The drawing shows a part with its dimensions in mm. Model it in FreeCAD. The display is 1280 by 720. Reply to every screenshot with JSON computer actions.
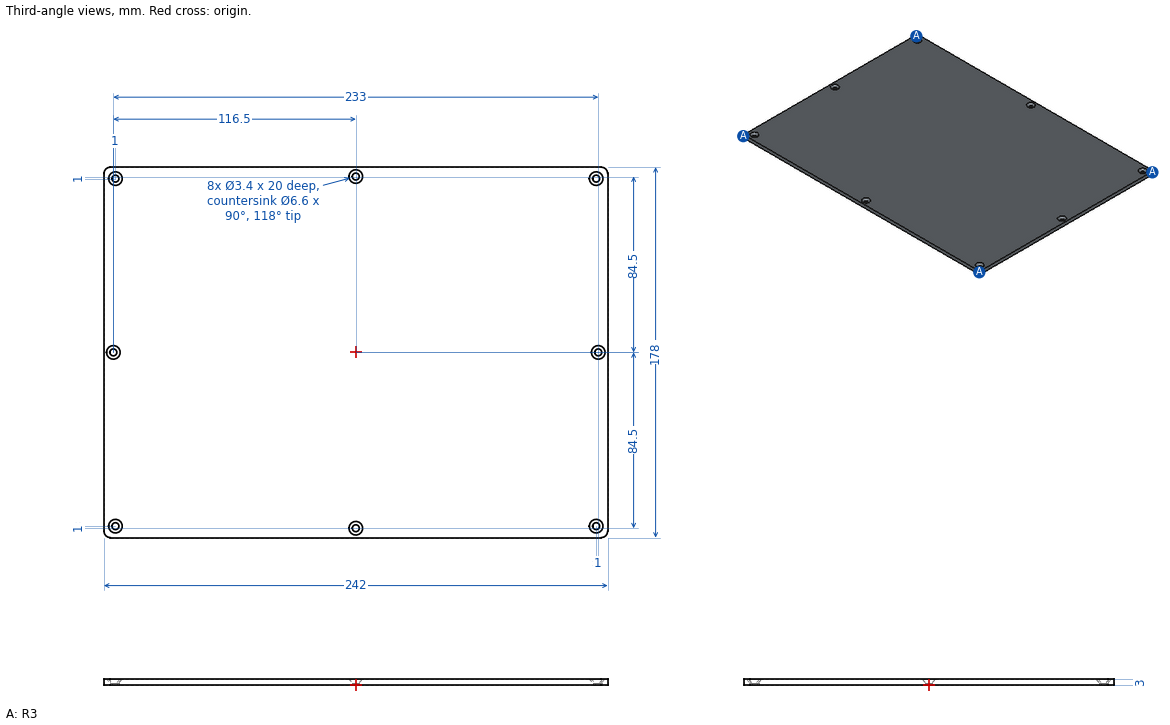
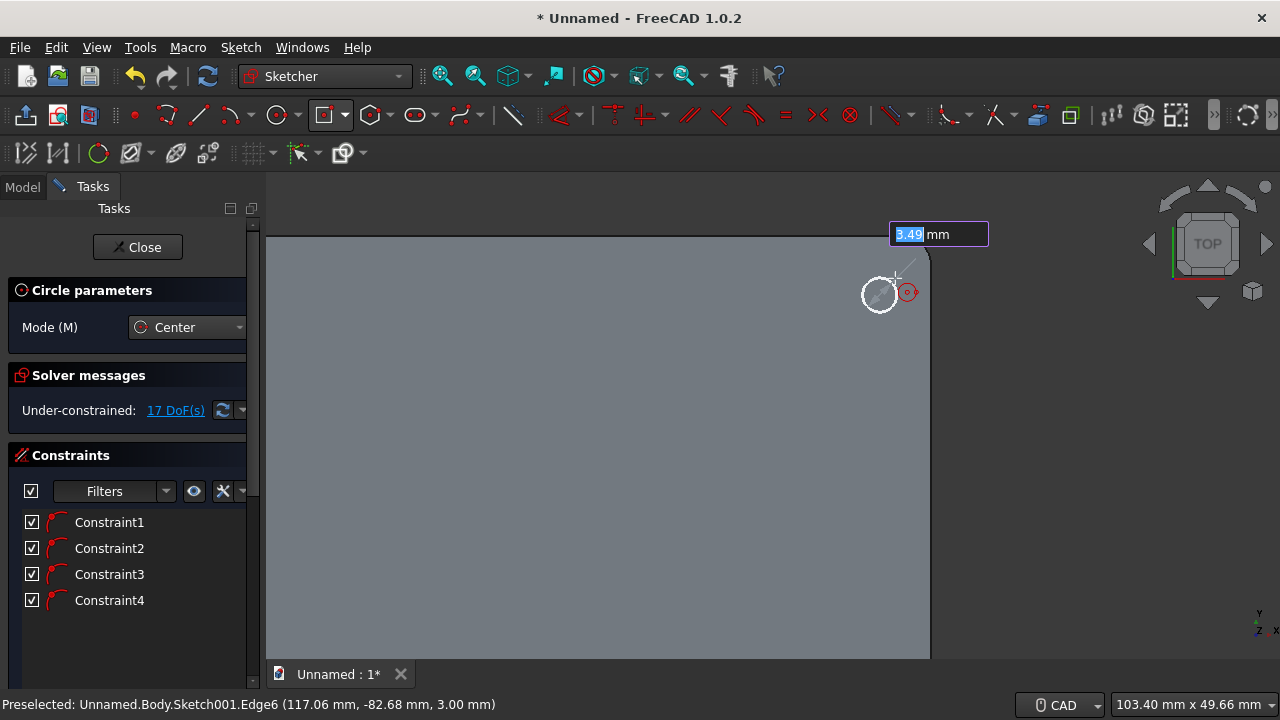
{"action": "left_click", "coordinate": [889, 278]}
{"action": "key", "text": "Escape"}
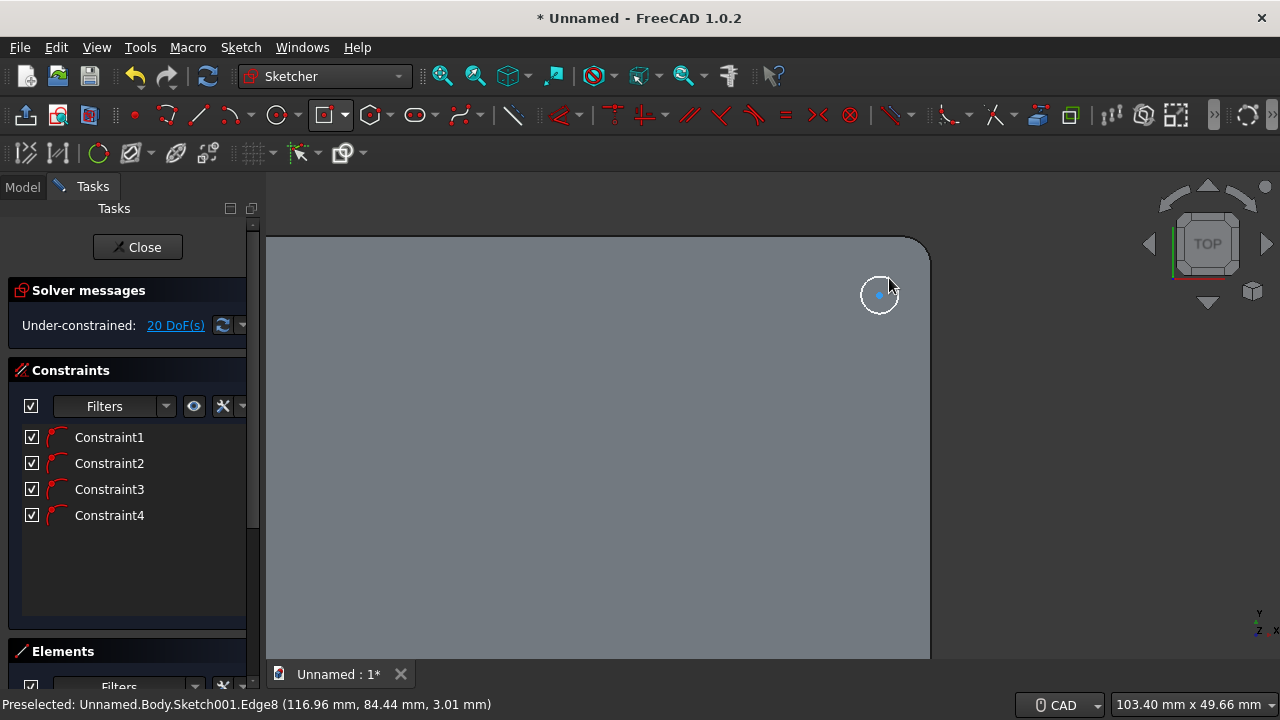
{"action": "scroll", "coordinate": [895, 278], "scroll_direction": "down", "scroll_amount": 9}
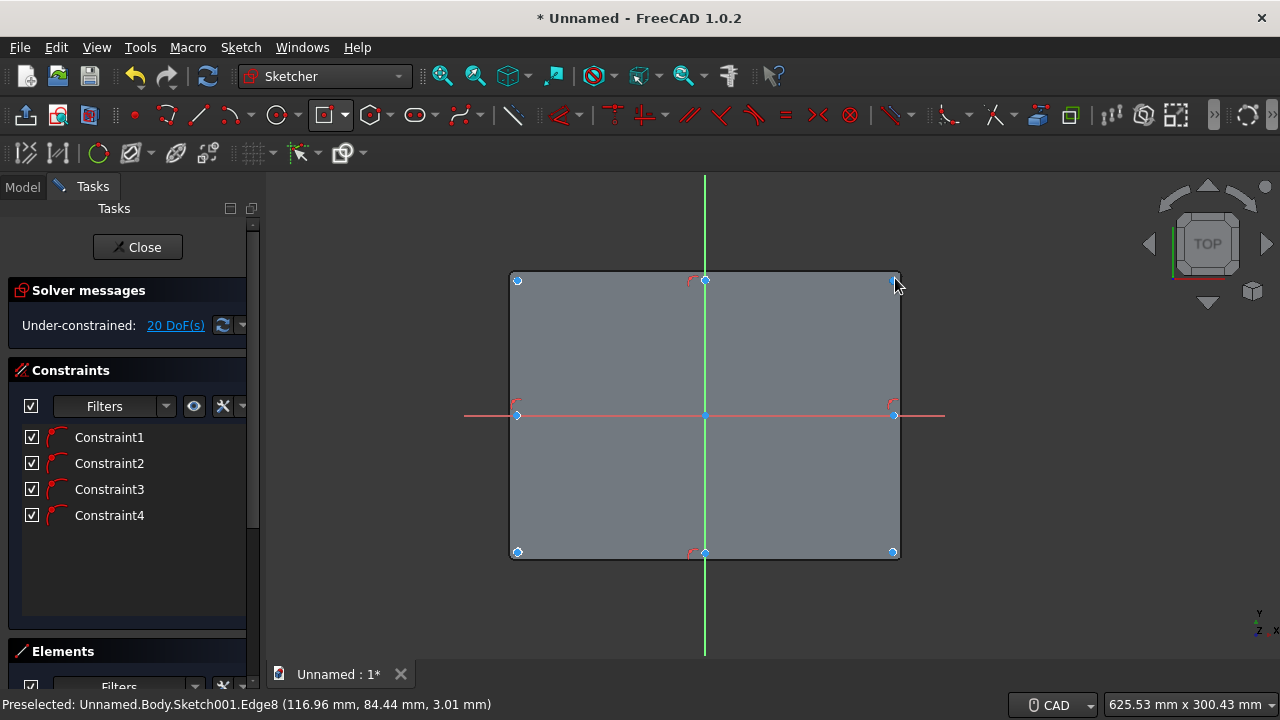
{"action": "scroll", "coordinate": [708, 278], "scroll_direction": "up", "scroll_amount": 9}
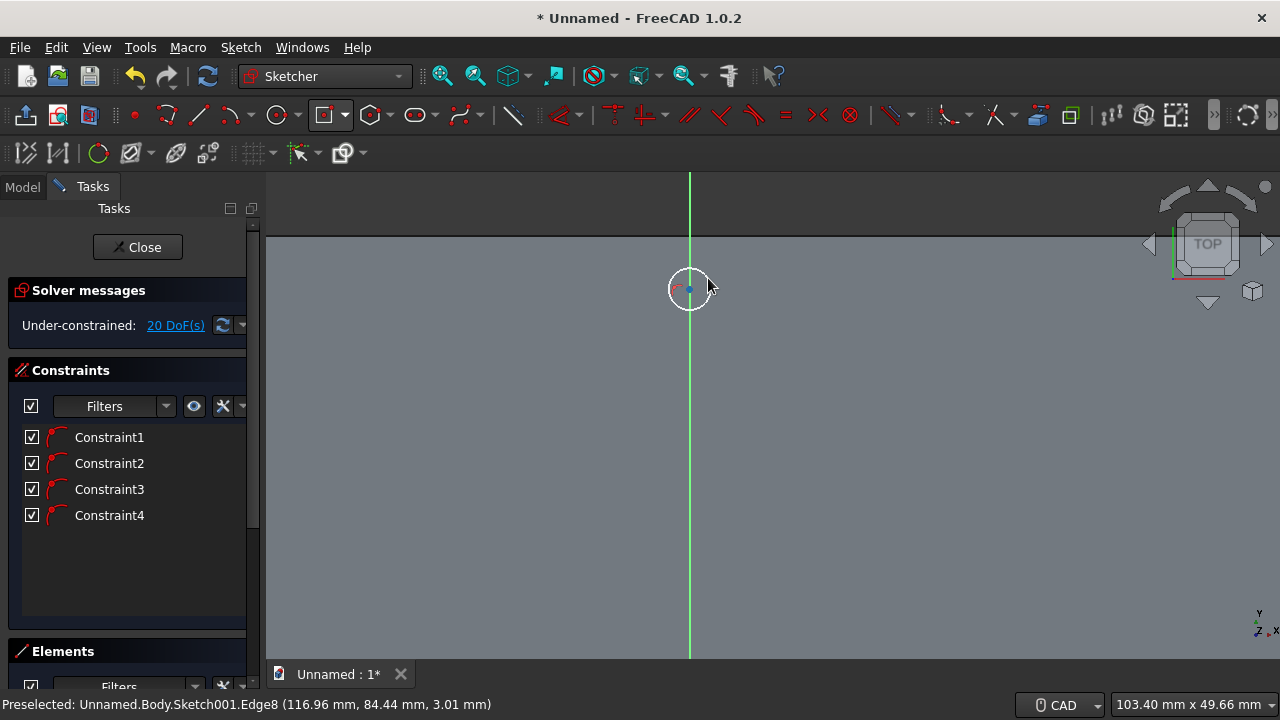
{"action": "left_click", "coordinate": [704, 274]}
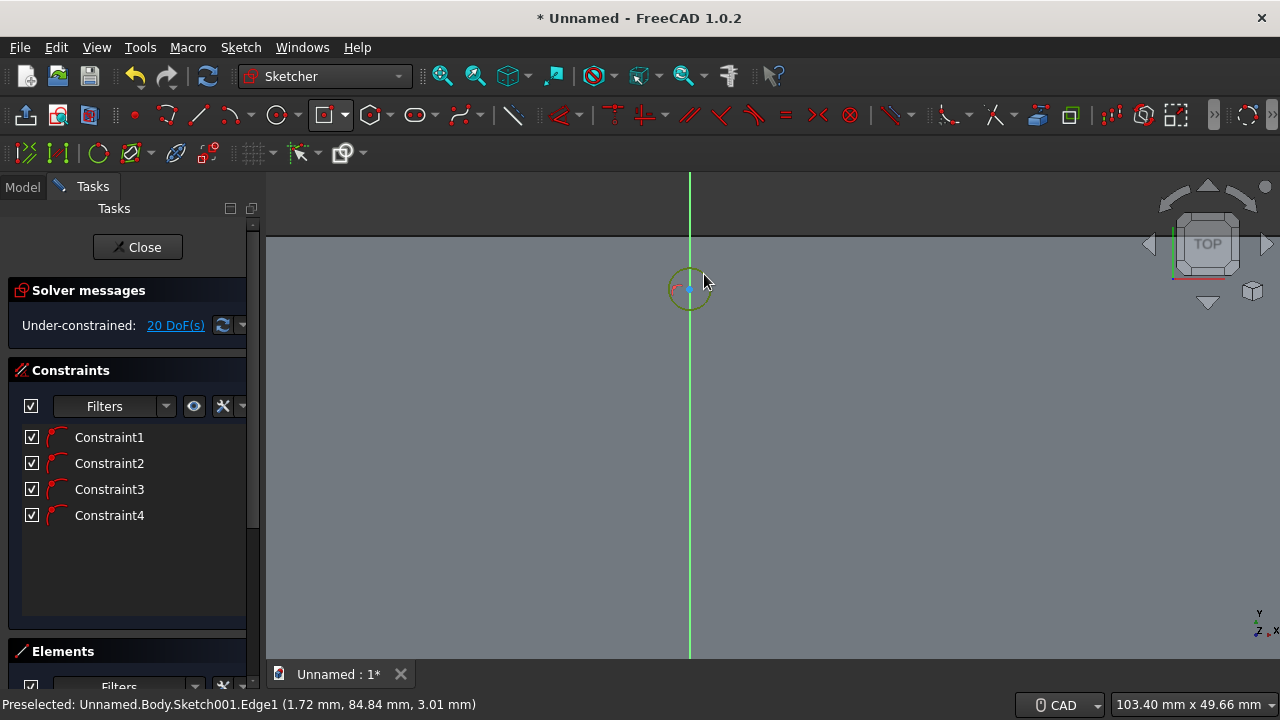
{"action": "scroll", "coordinate": [707, 278], "scroll_direction": "down", "scroll_amount": 9}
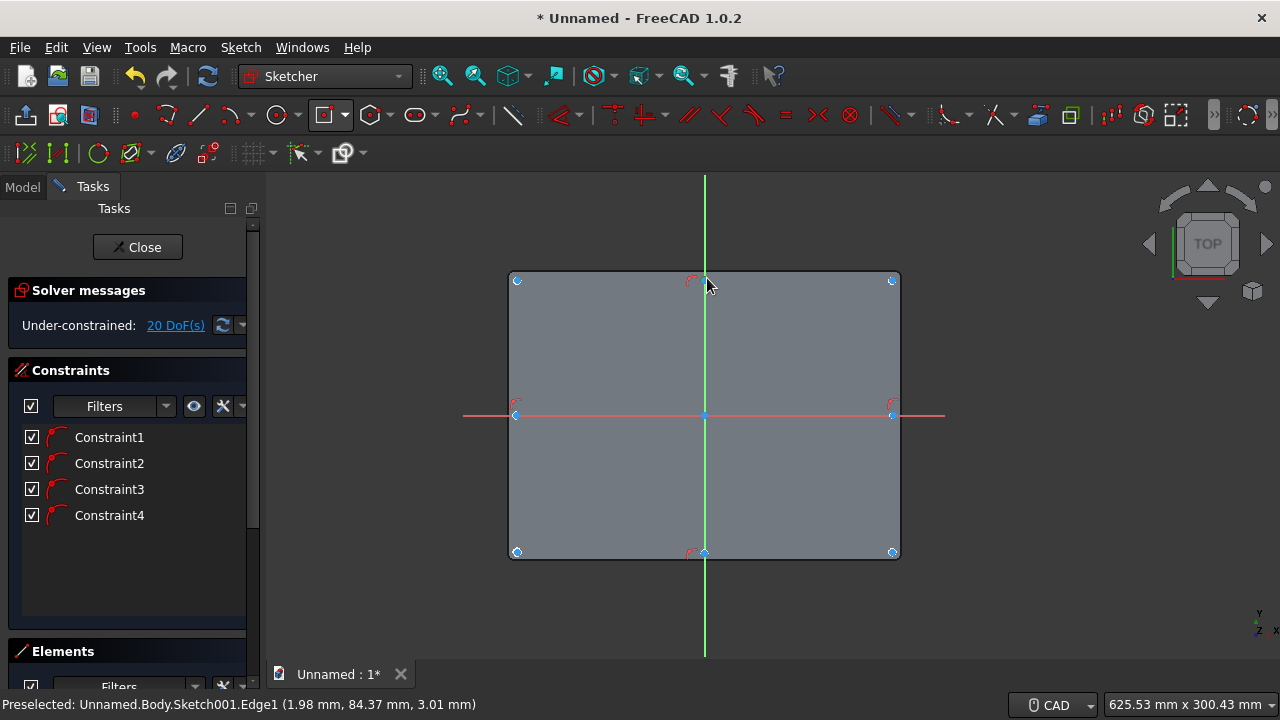
{"action": "scroll", "coordinate": [518, 413], "scroll_direction": "up", "scroll_amount": 10}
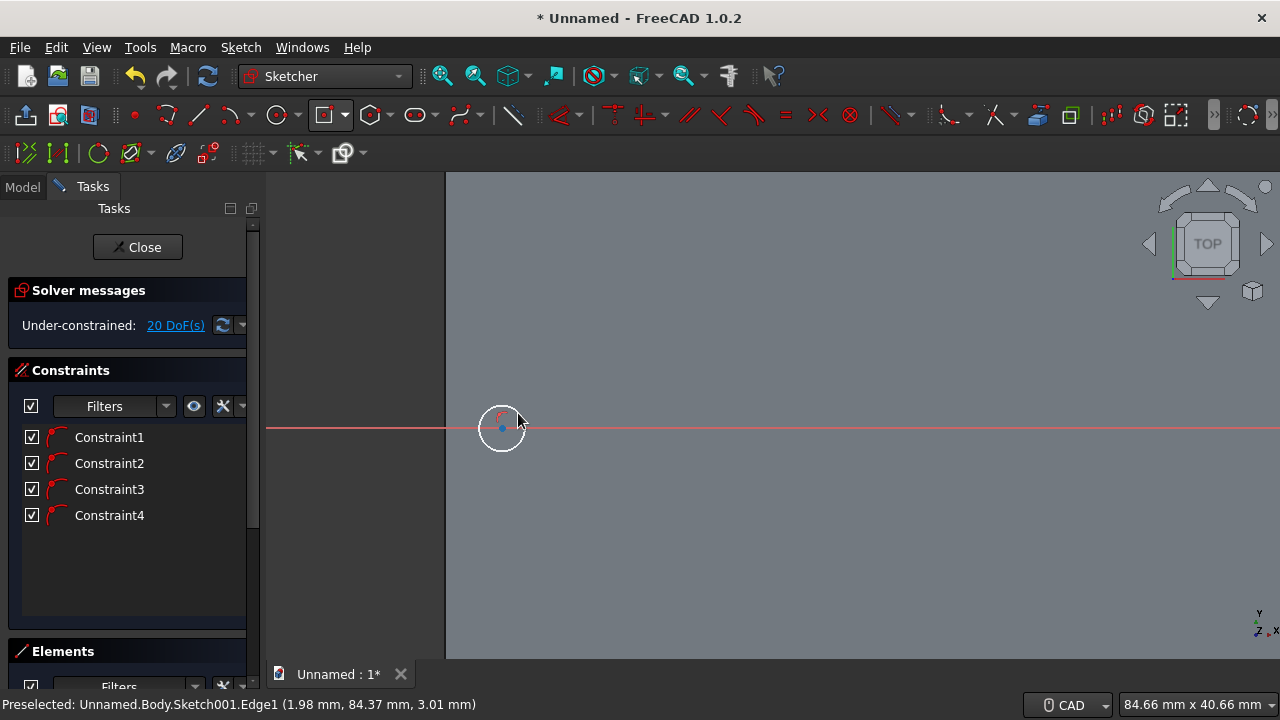
{"action": "left_click", "coordinate": [518, 412]}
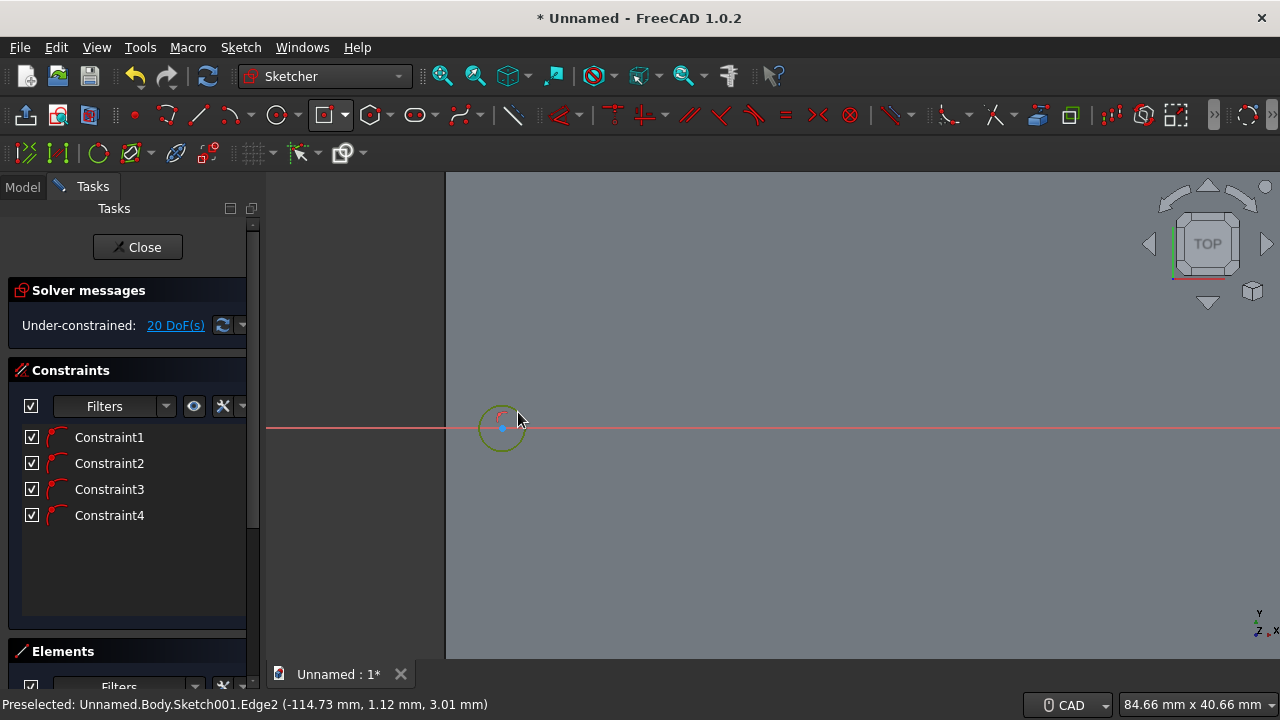
{"action": "scroll", "coordinate": [518, 413], "scroll_direction": "down", "scroll_amount": 10}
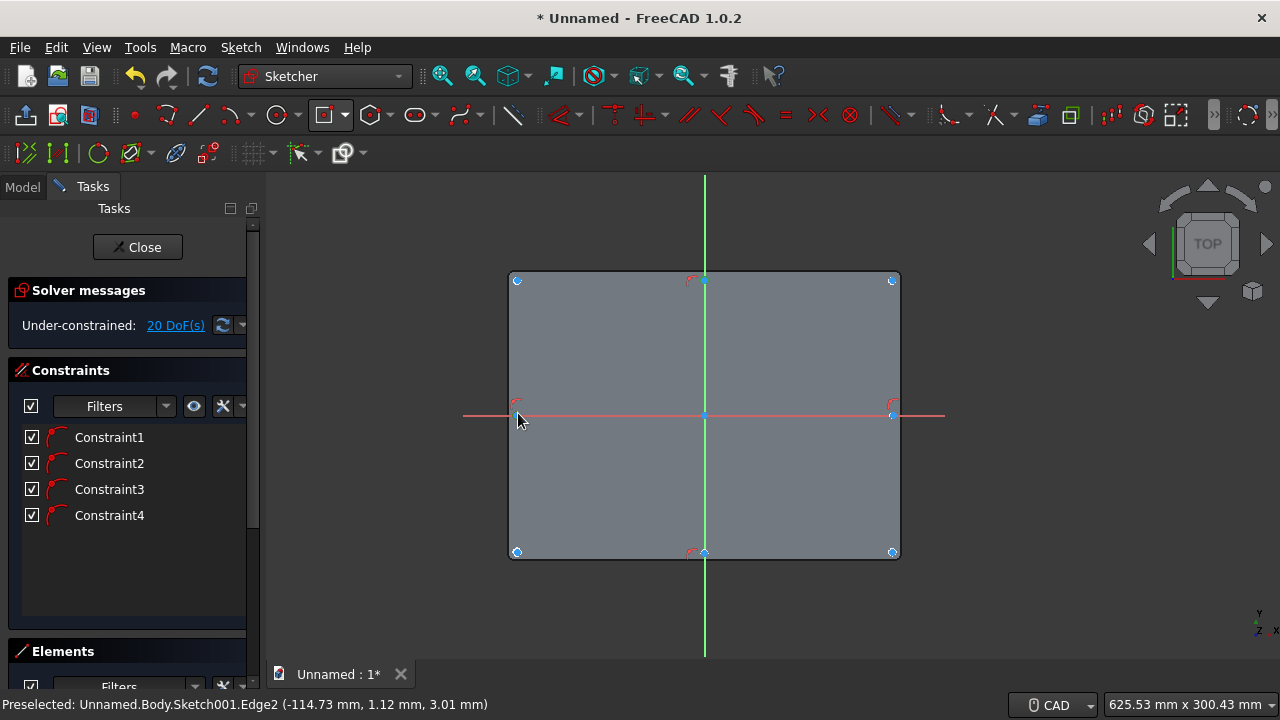
{"action": "scroll", "coordinate": [707, 551], "scroll_direction": "up", "scroll_amount": 10}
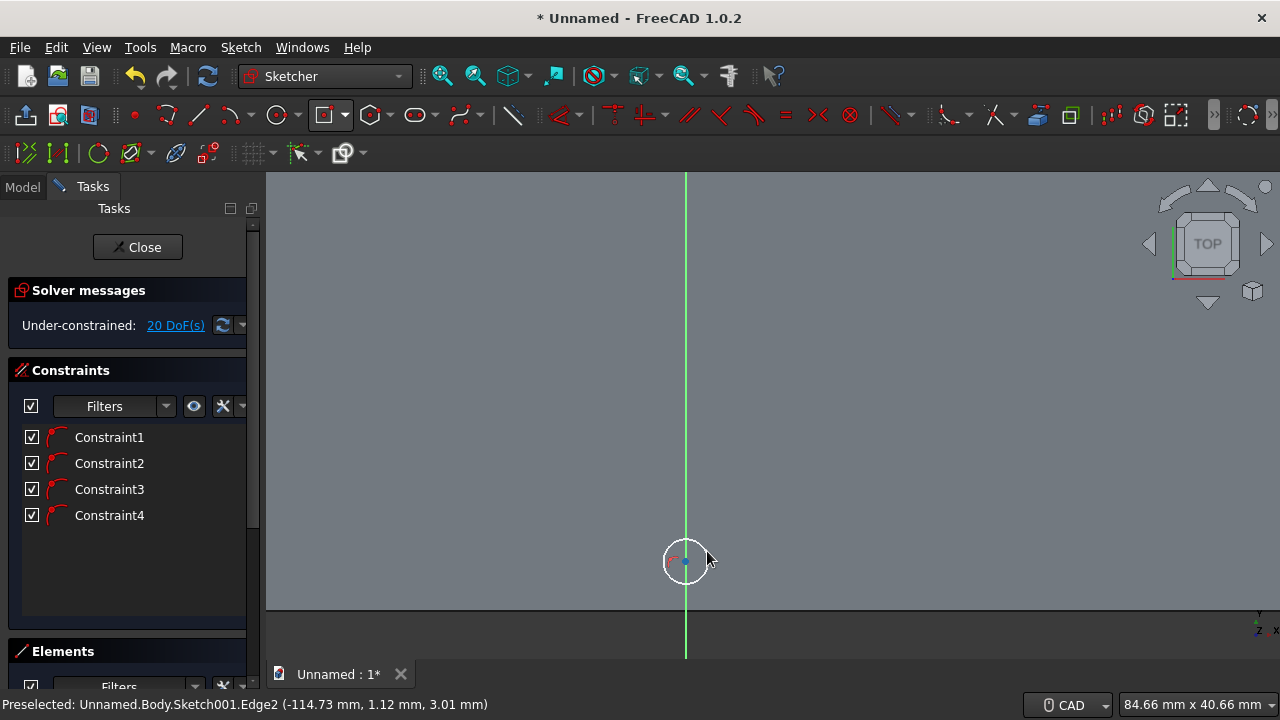
{"action": "left_click", "coordinate": [702, 546]}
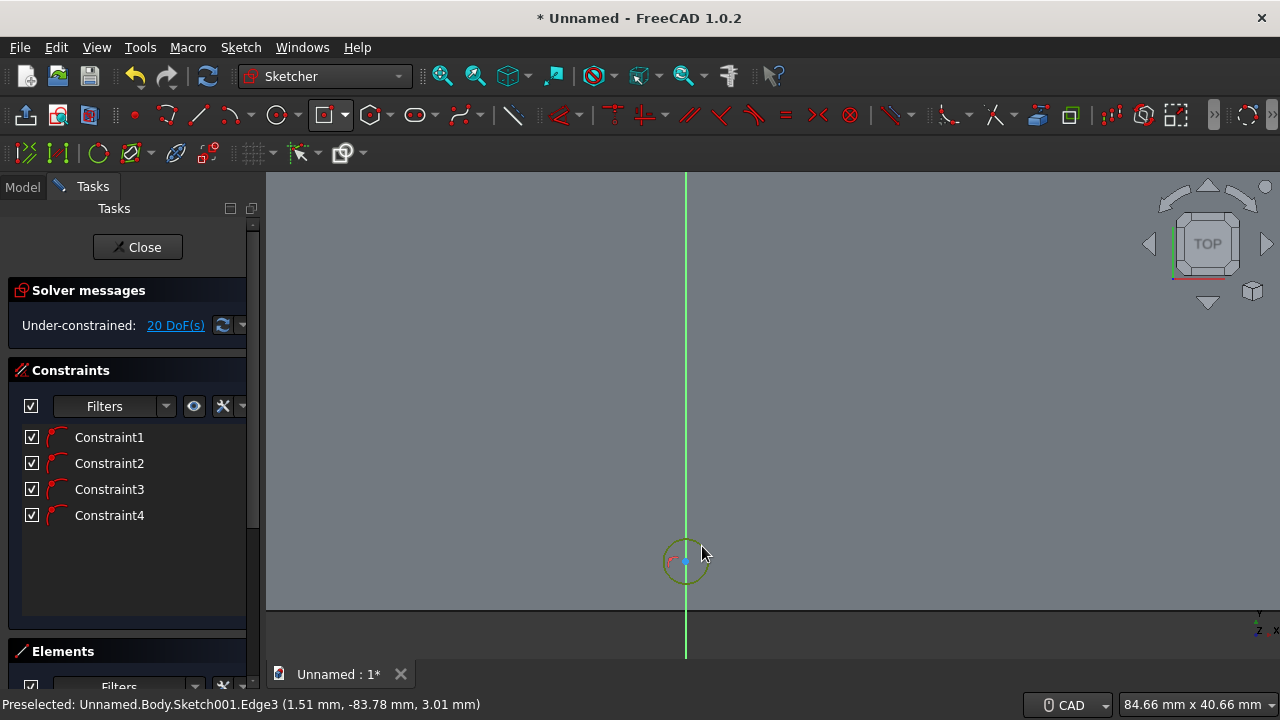
{"action": "scroll", "coordinate": [707, 552], "scroll_direction": "down", "scroll_amount": 10}